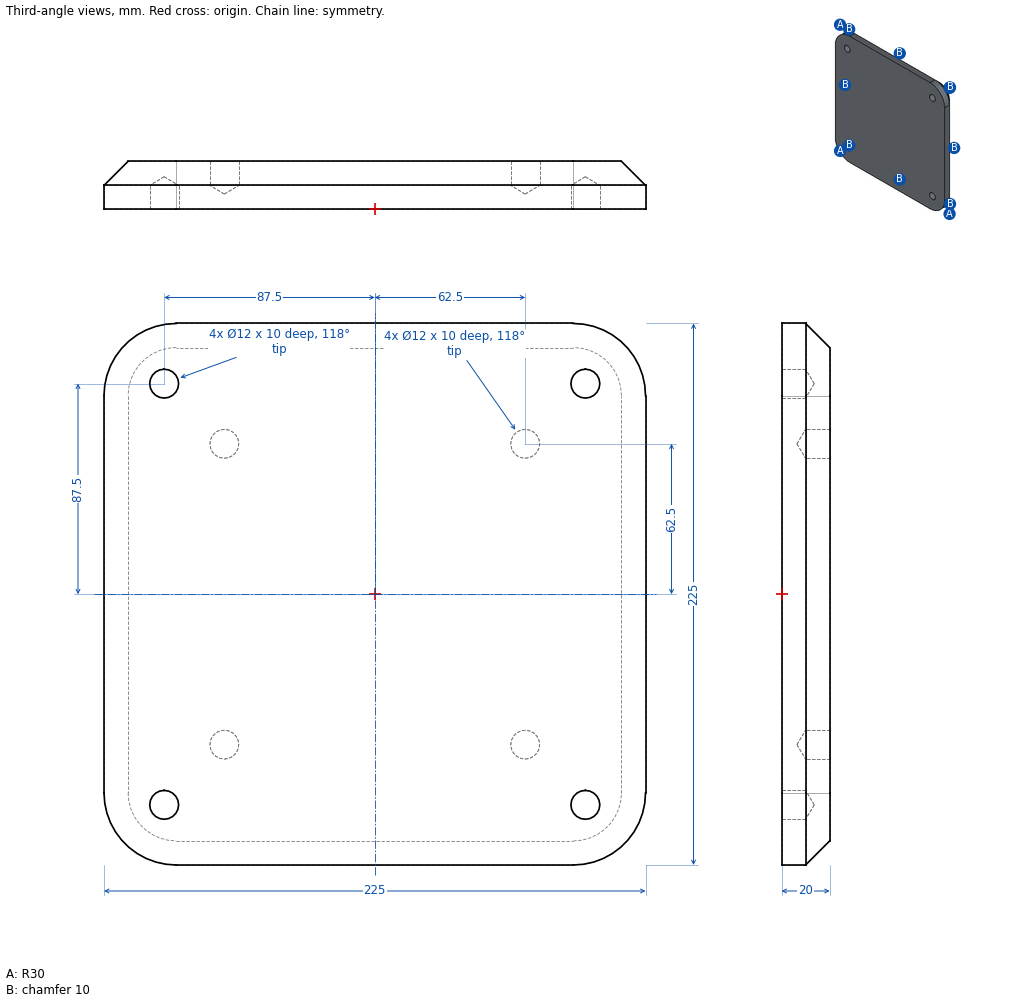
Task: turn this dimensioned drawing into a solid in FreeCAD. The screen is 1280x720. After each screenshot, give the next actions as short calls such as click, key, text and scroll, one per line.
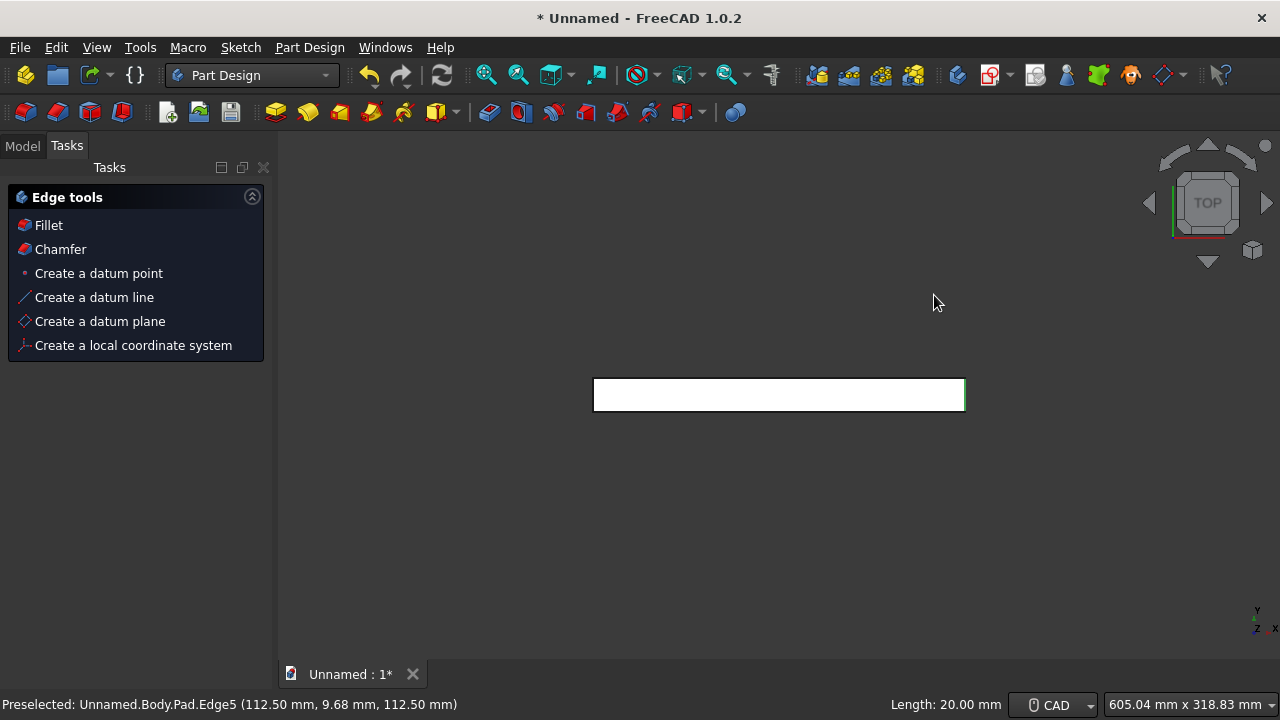
click(488, 76)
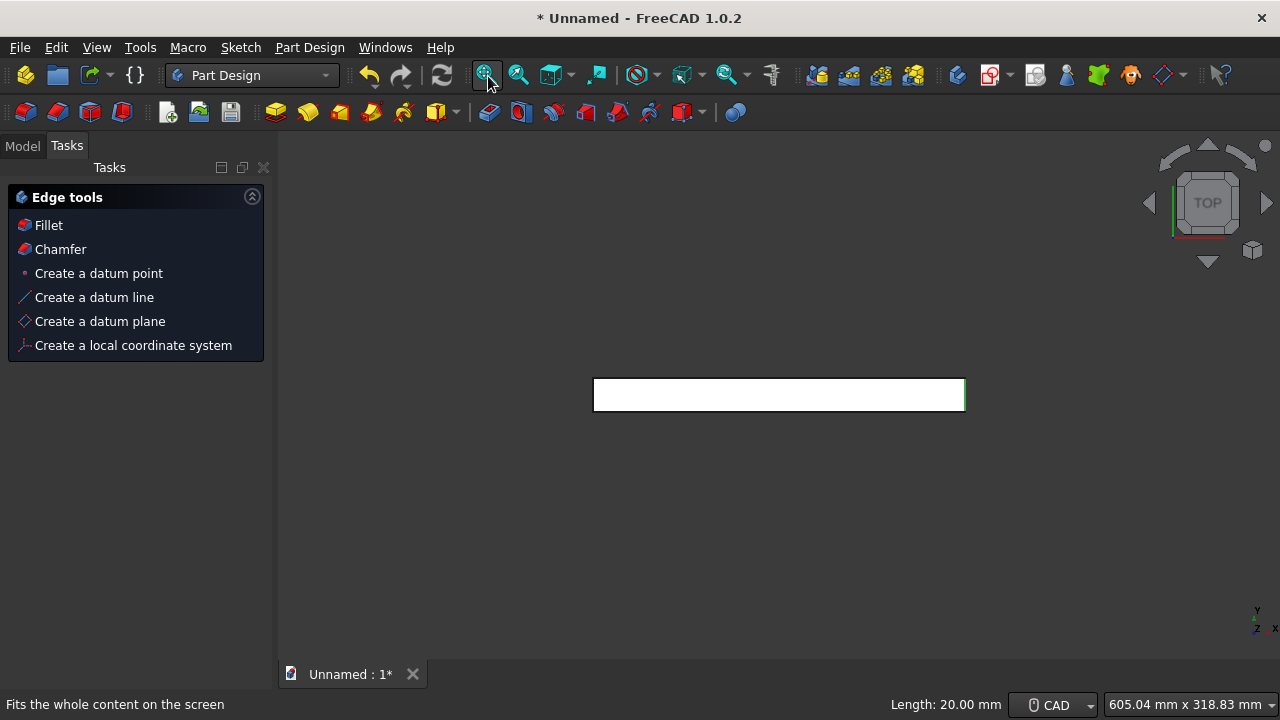
click(593, 394, ctrl)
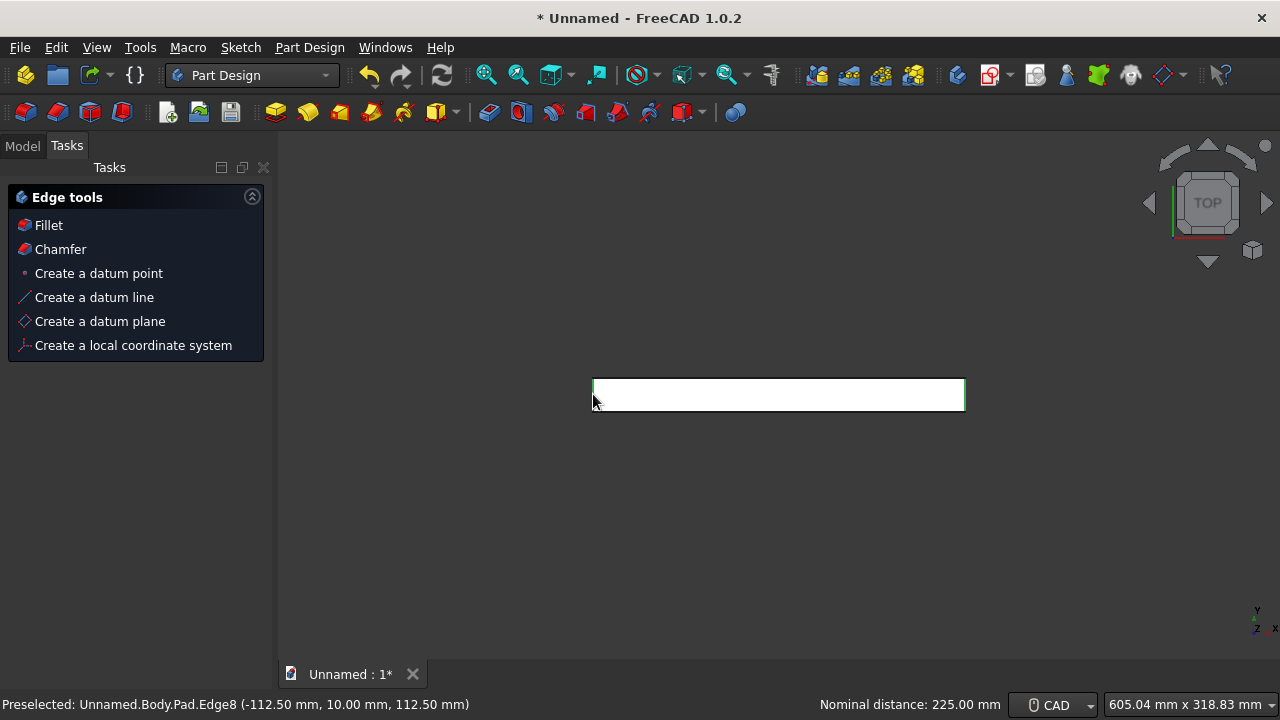
key(1)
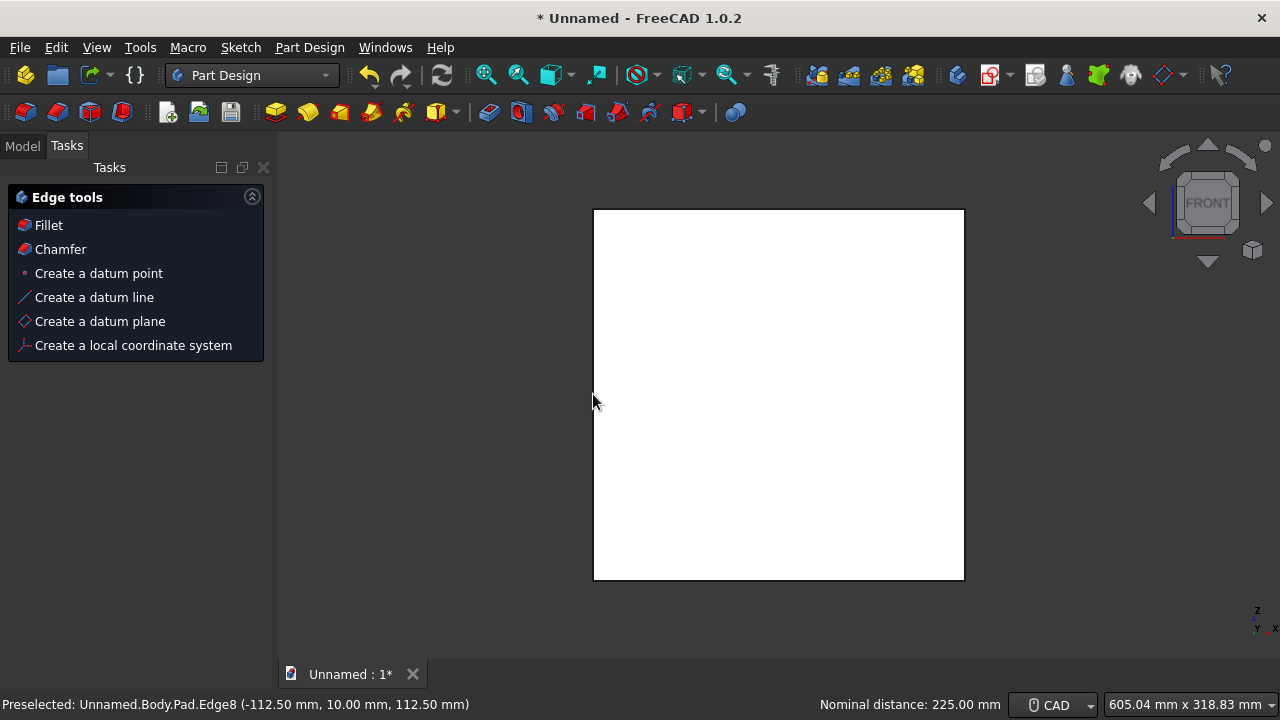
key(3)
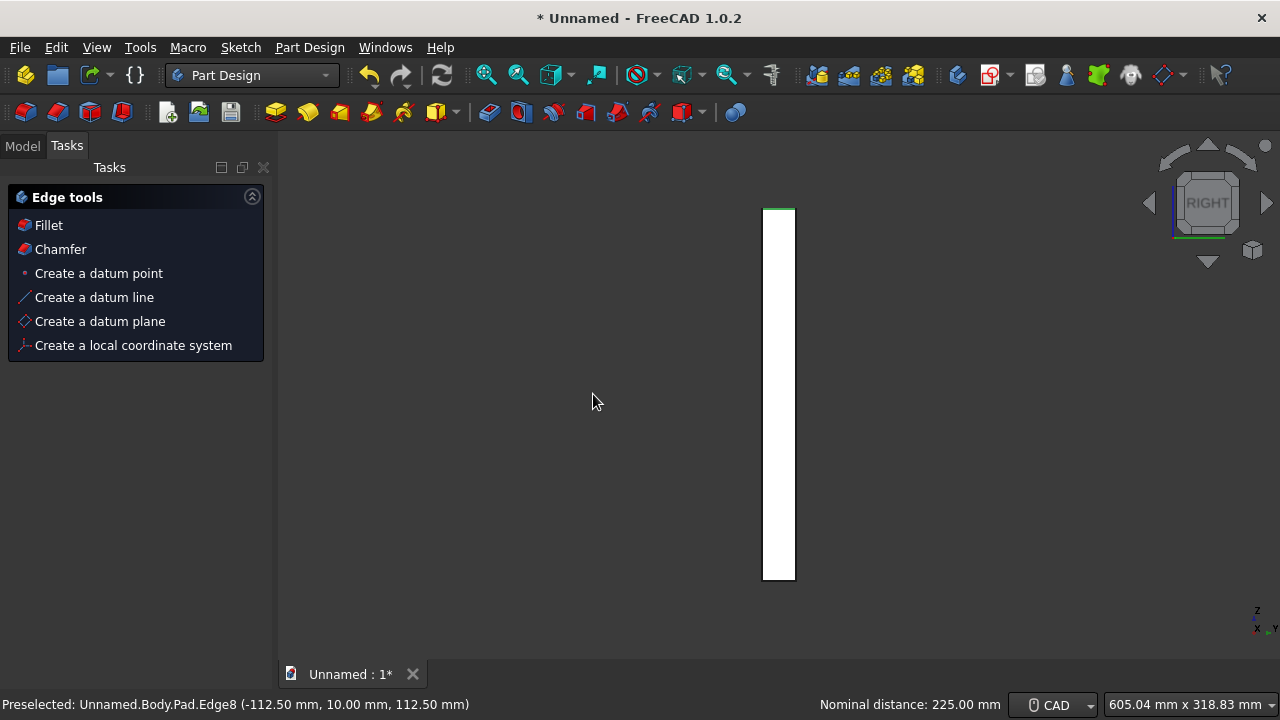
click(779, 580, ctrl)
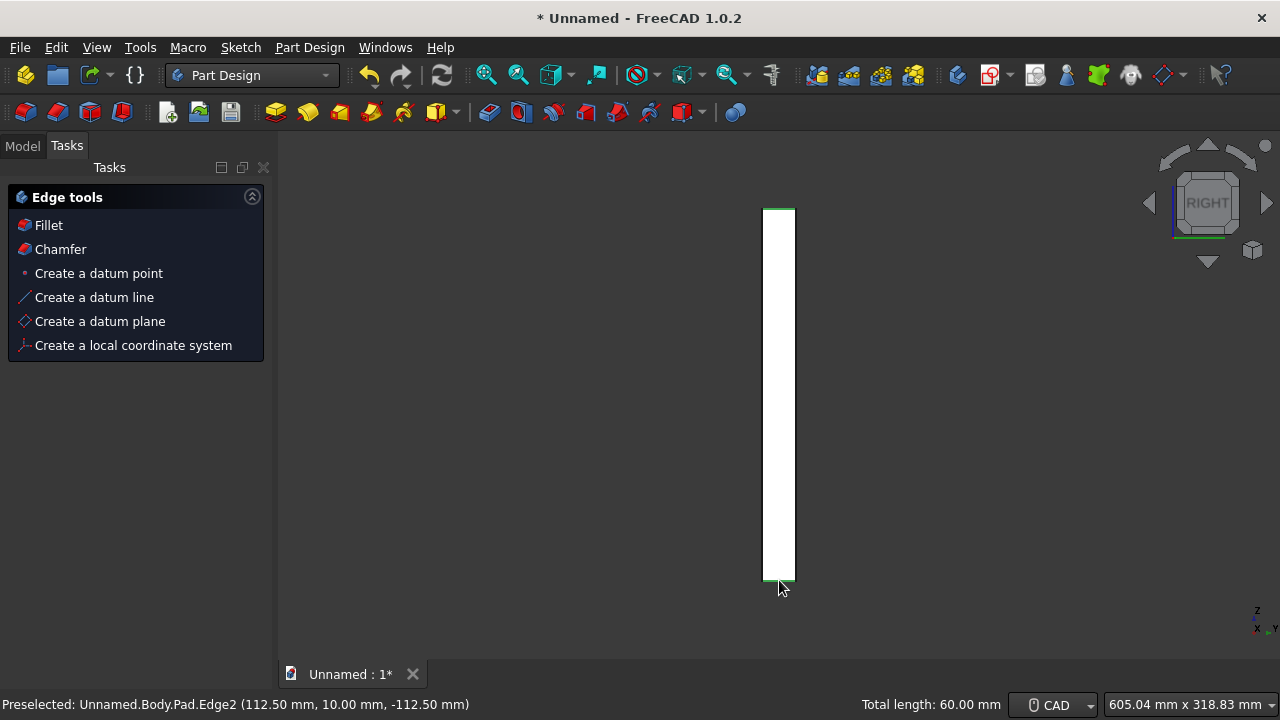
key(5)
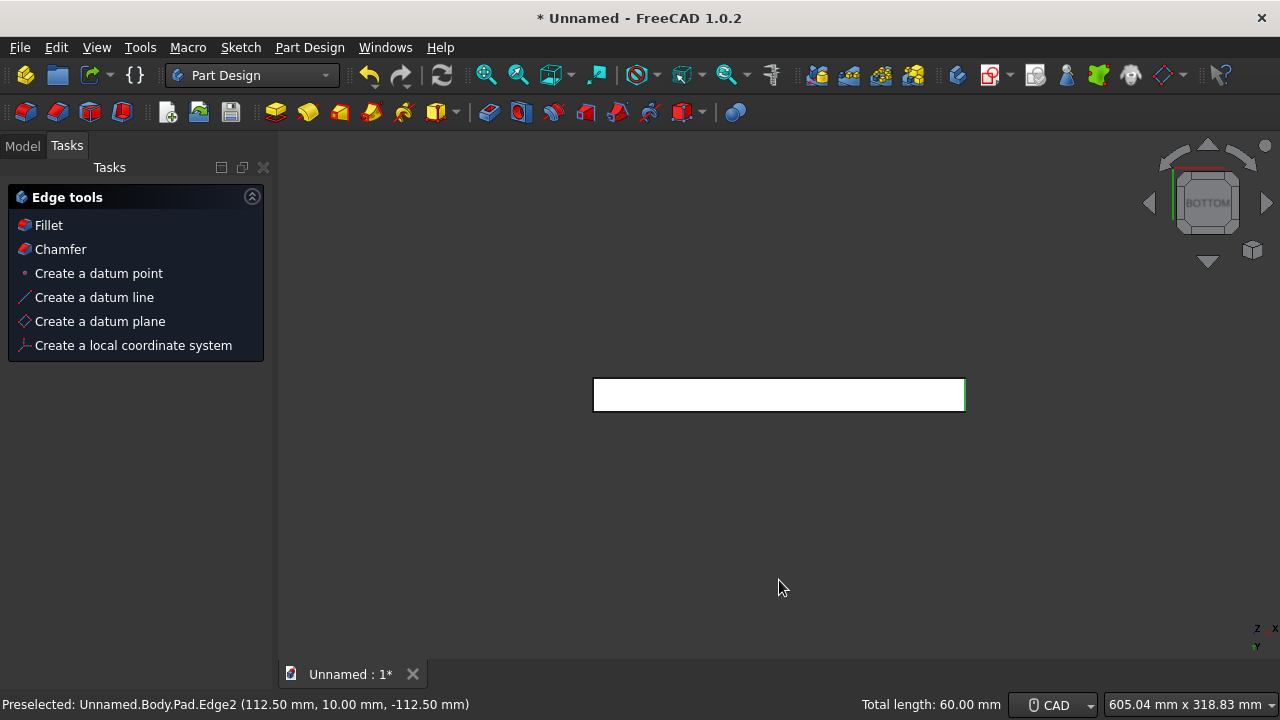
key(v)
key(f)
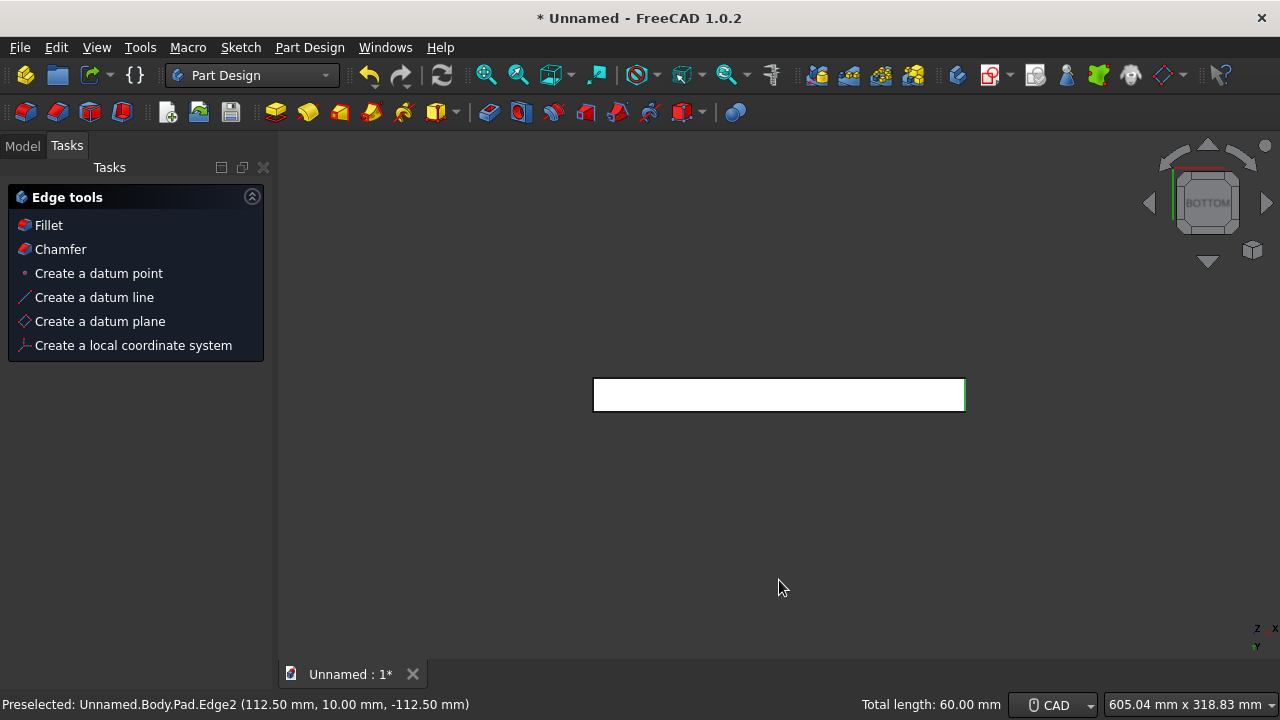
click(593, 394, ctrl)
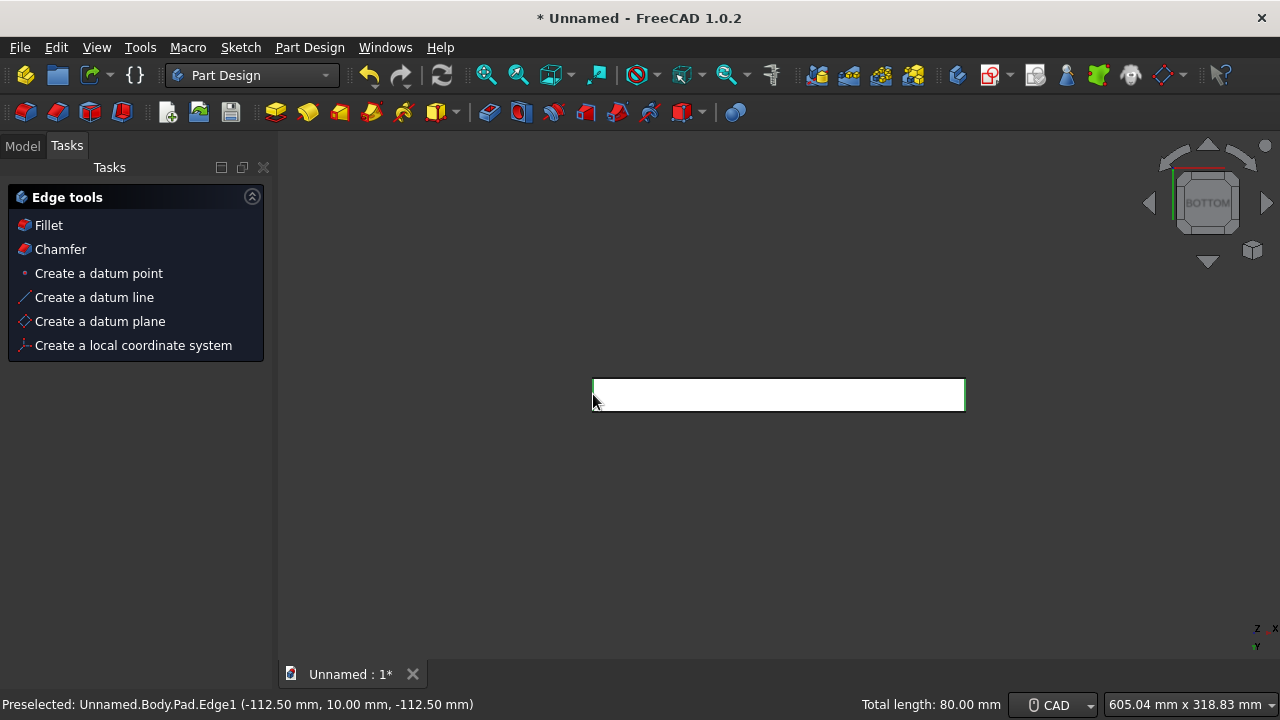
click(26, 112)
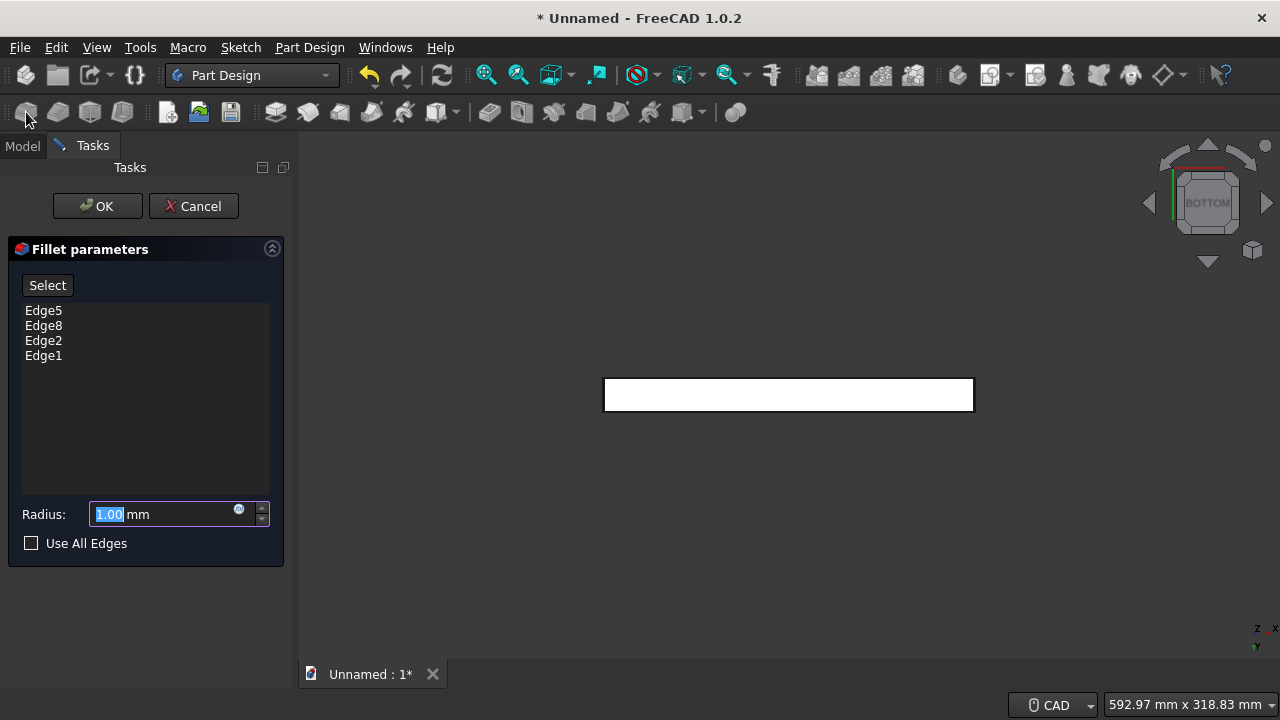
text(30)
key(Tab)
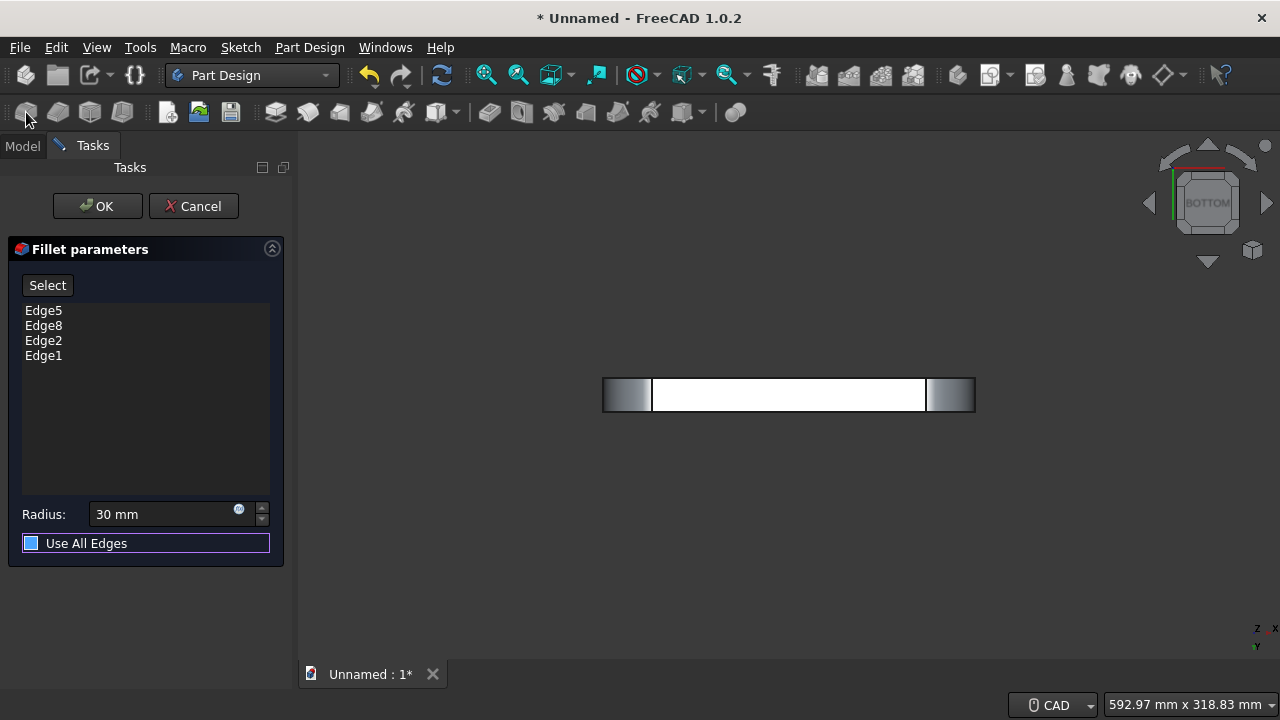
click(98, 206)